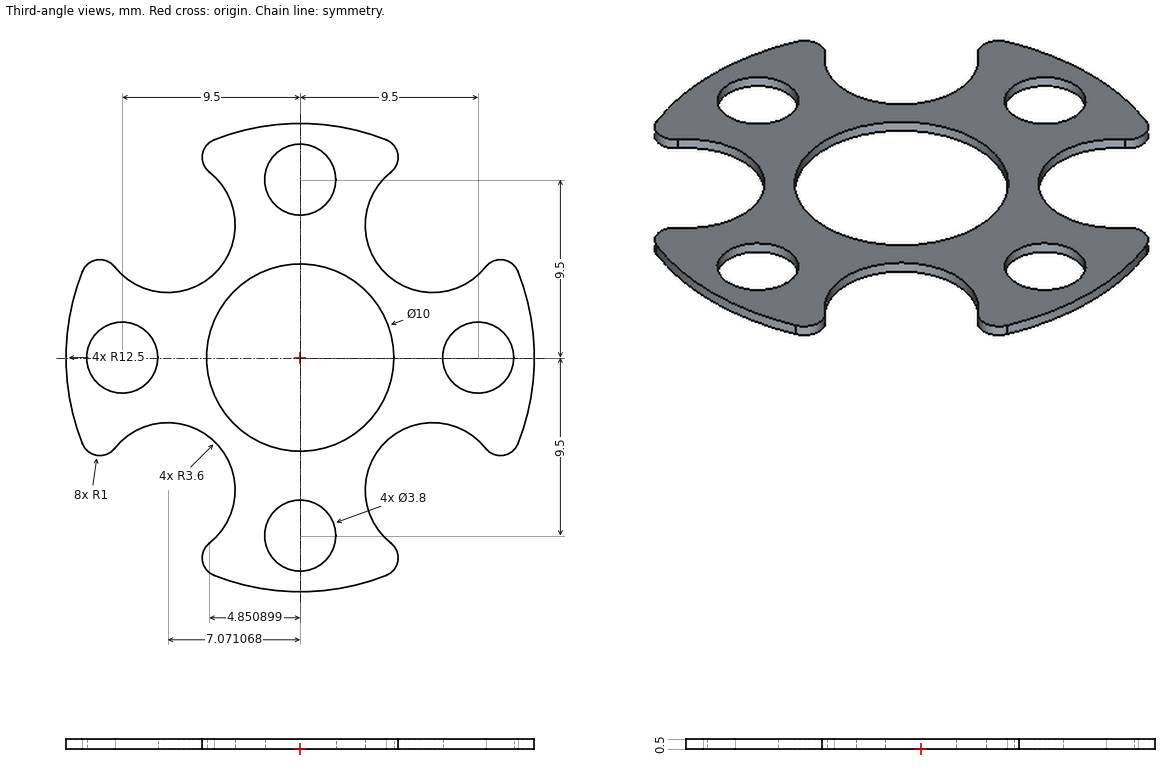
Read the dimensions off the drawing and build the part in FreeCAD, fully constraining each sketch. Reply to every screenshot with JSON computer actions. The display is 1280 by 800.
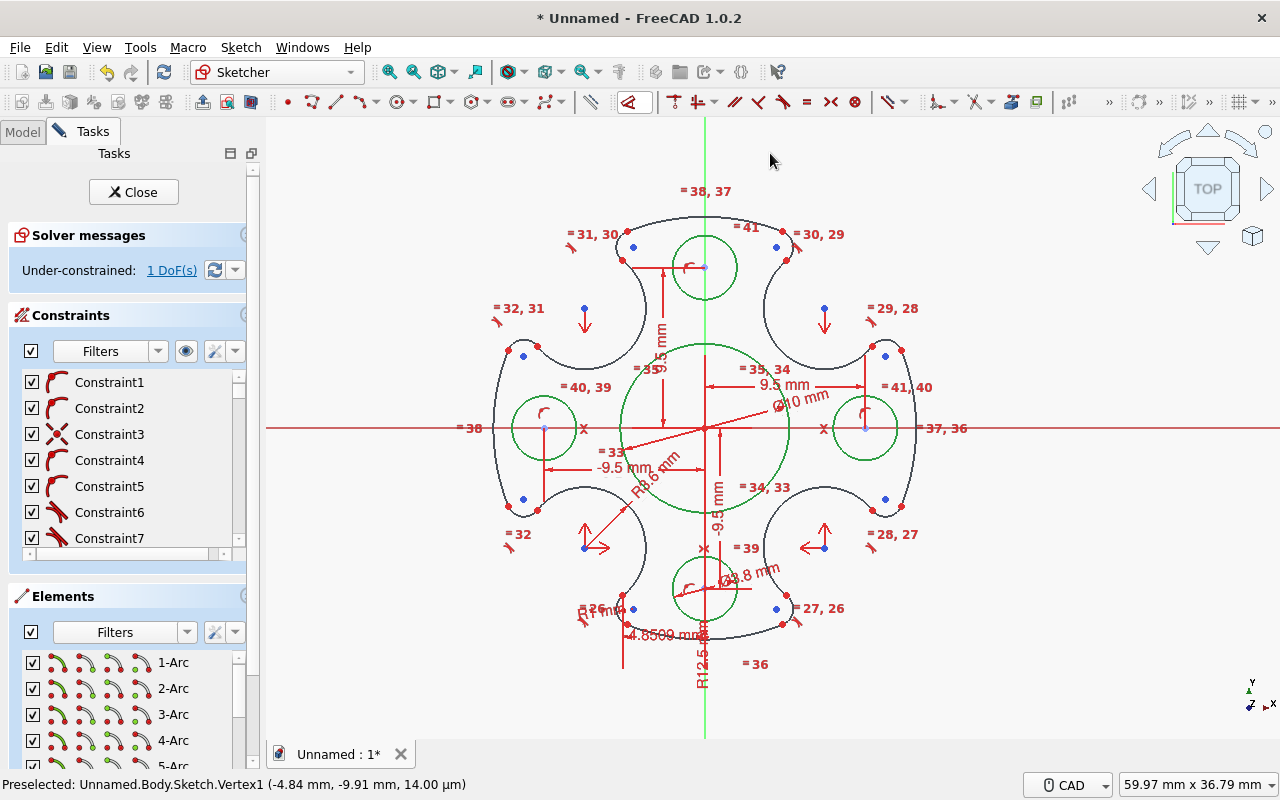
{"action": "left_click", "coordinate": [585, 548]}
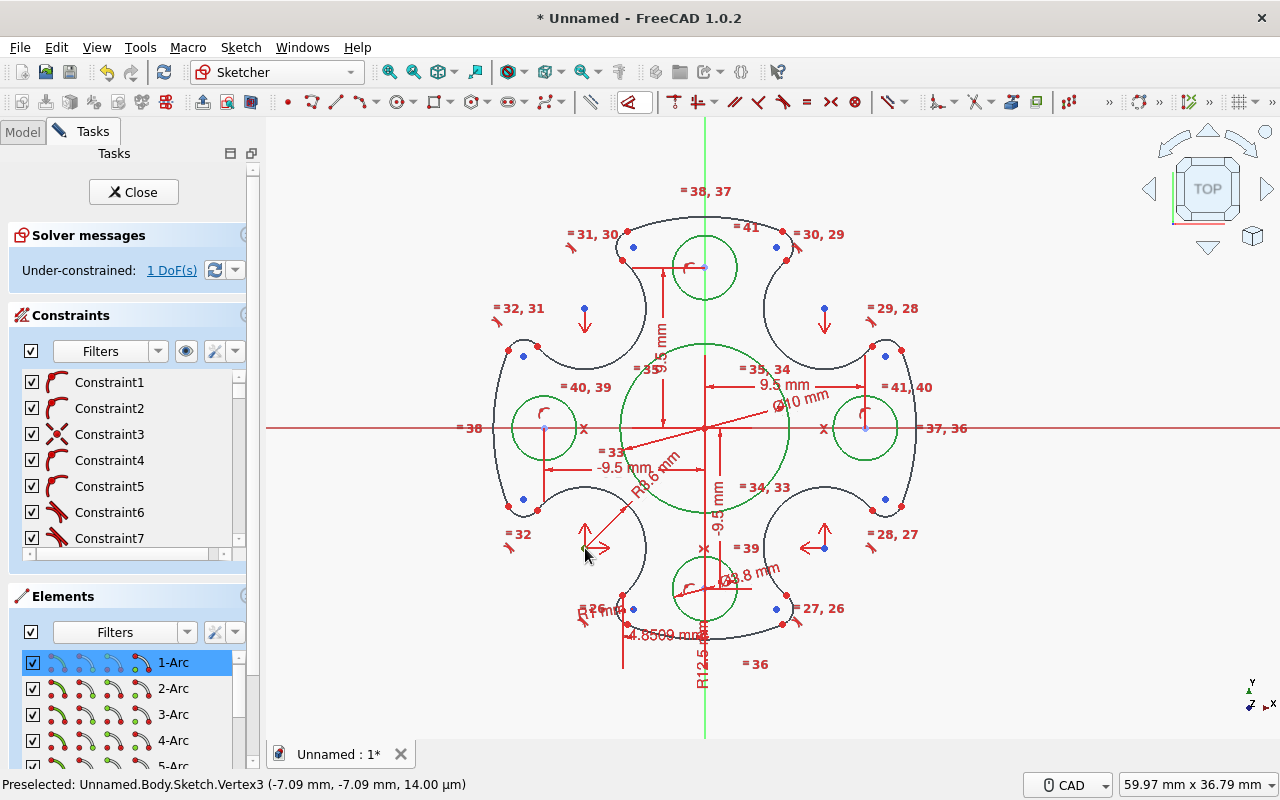
{"action": "left_click", "coordinate": [646, 102]}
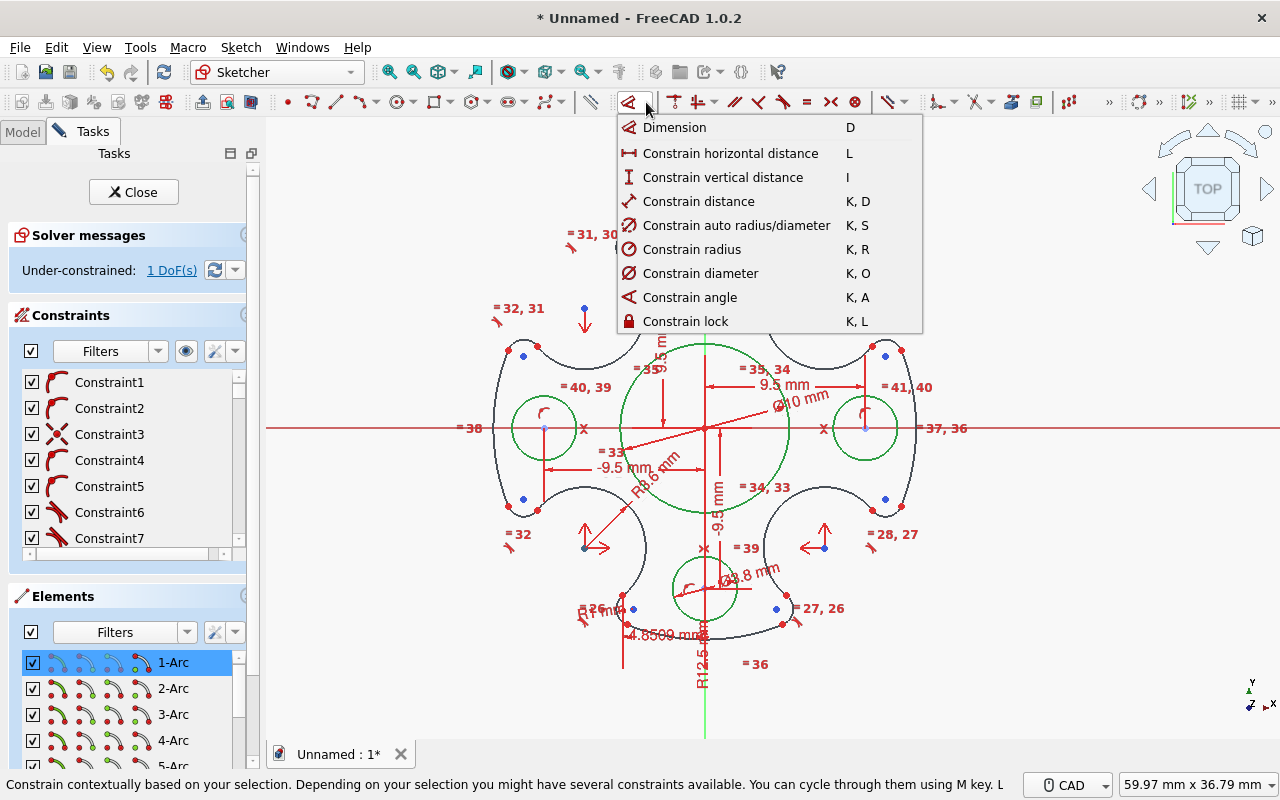
{"action": "left_click", "coordinate": [770, 153]}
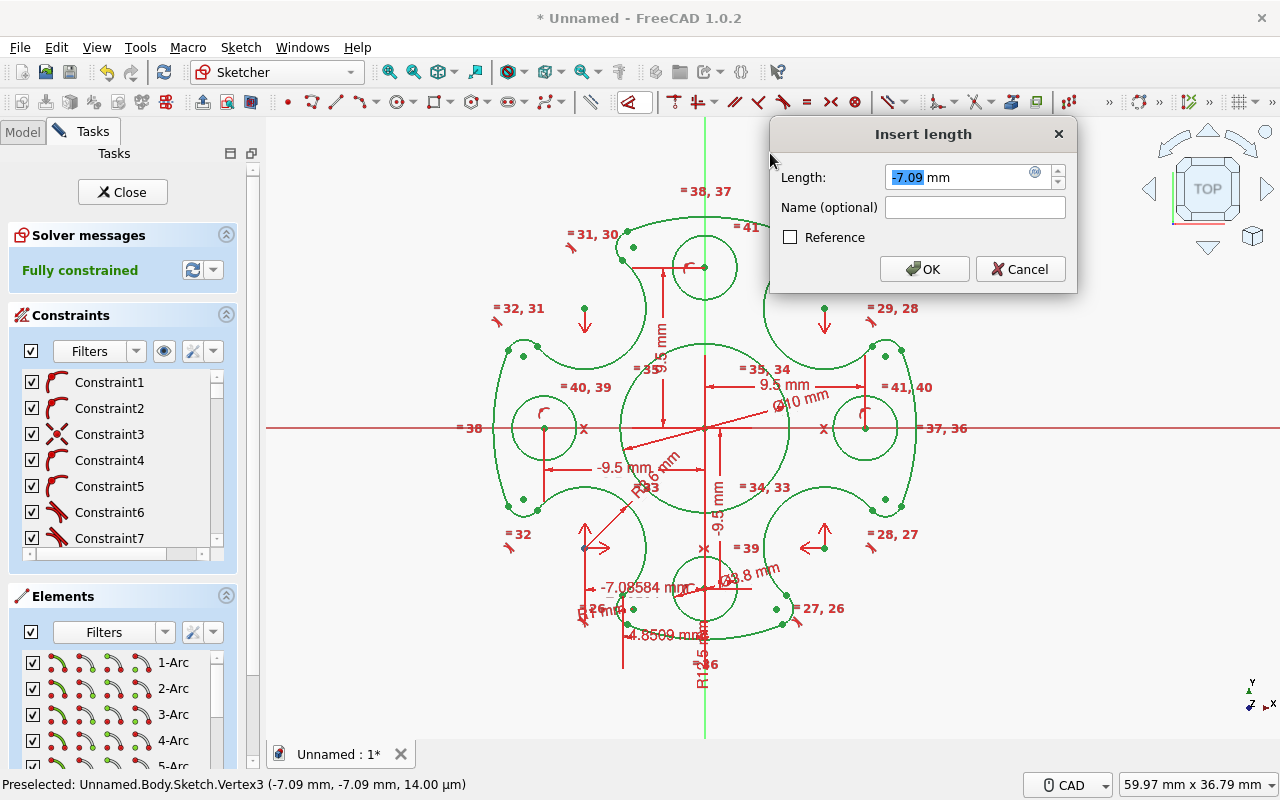
{"action": "type", "text": "-7.071068"}
{"action": "key", "text": "Return"}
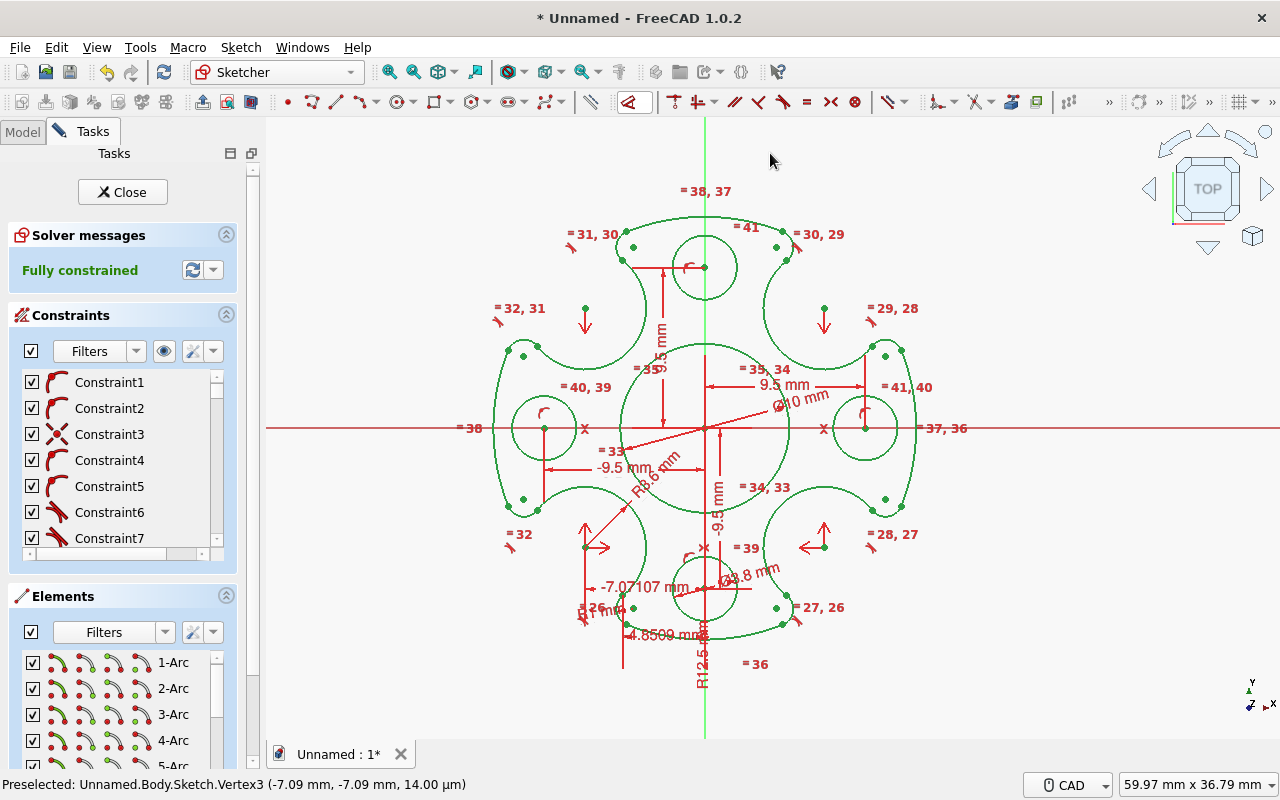
{"action": "left_click", "coordinate": [123, 192]}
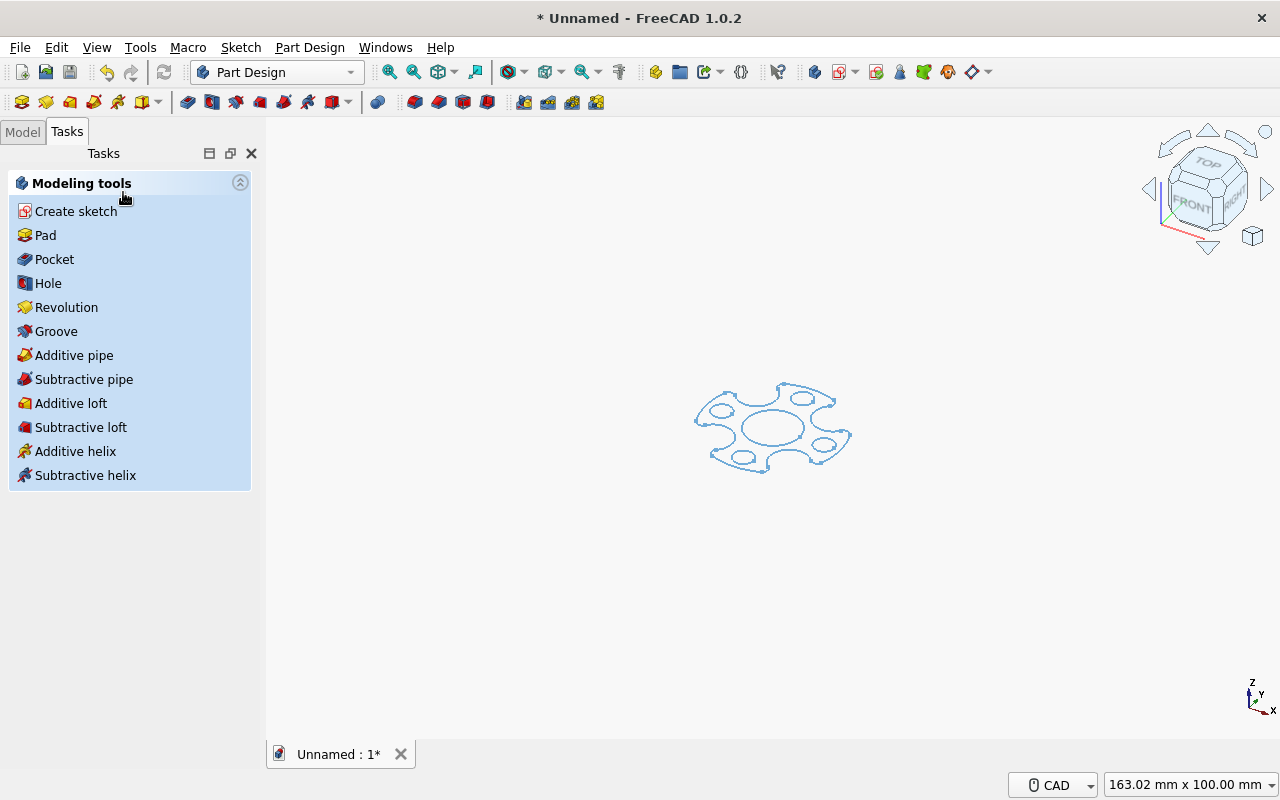
{"action": "left_click", "coordinate": [22, 102]}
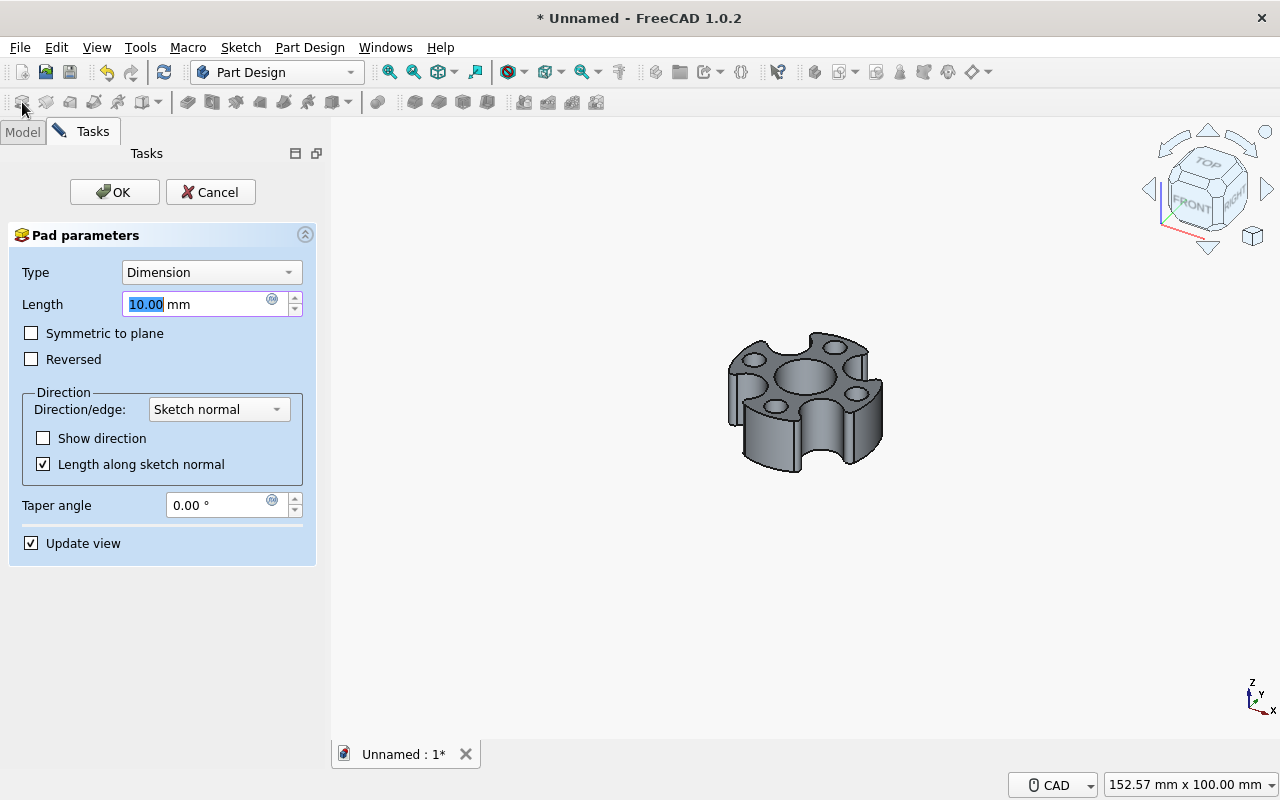
{"action": "type", "text": "0.5"}
{"action": "key", "text": "Tab"}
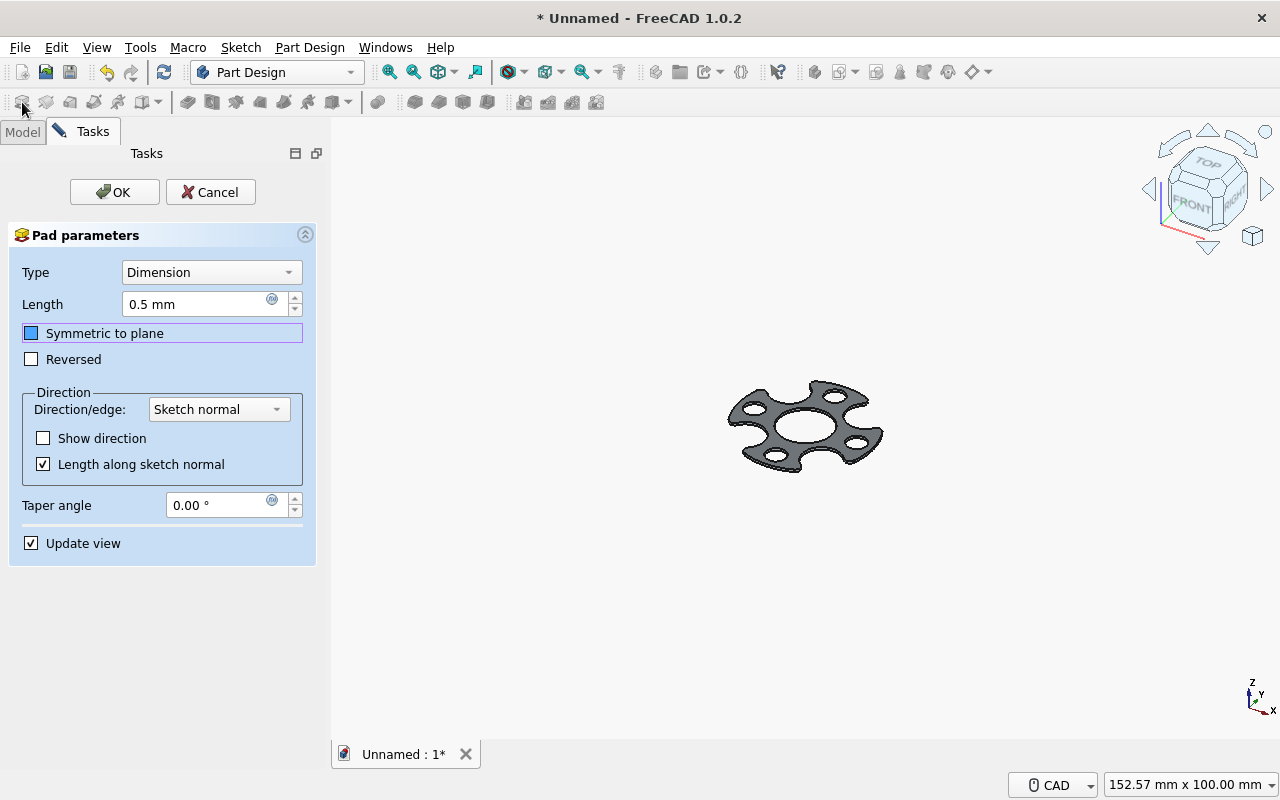
{"action": "left_click", "coordinate": [115, 192]}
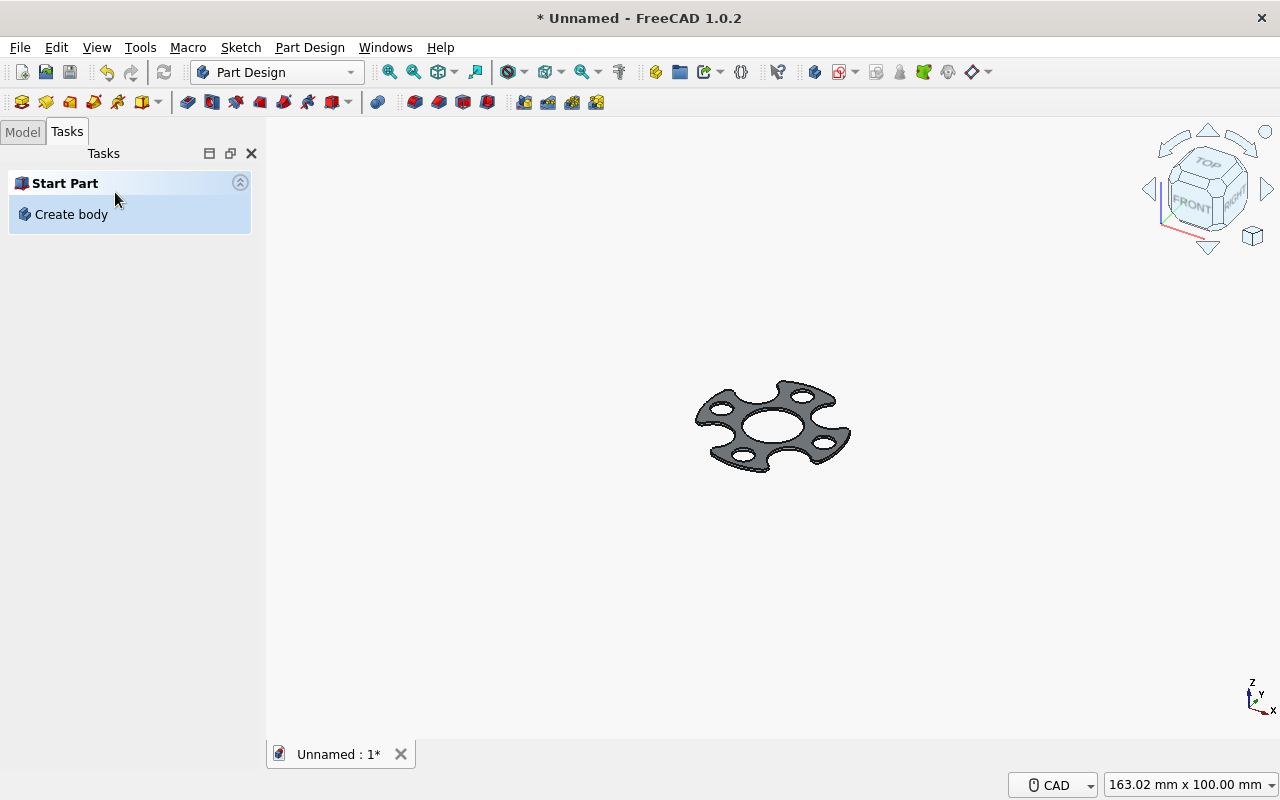
{"action": "key", "text": "0"}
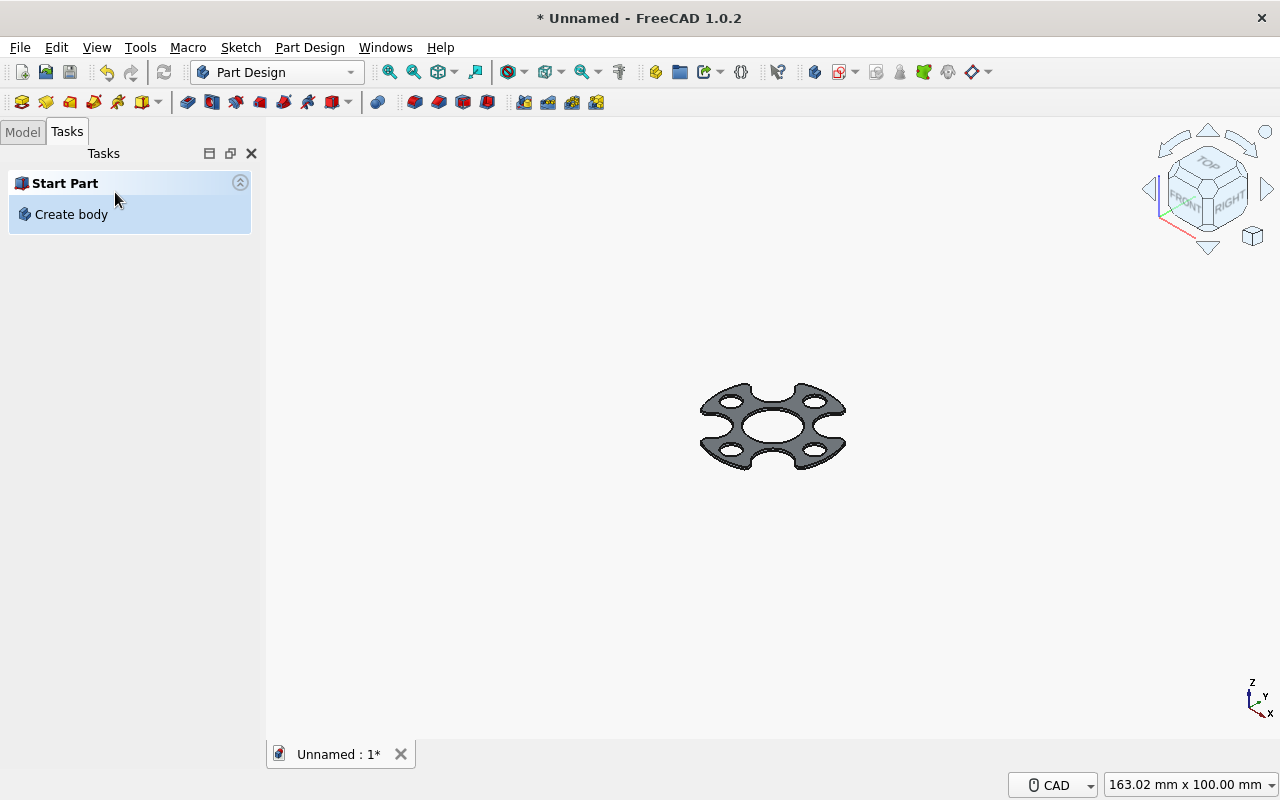
{"action": "key", "text": "v f"}